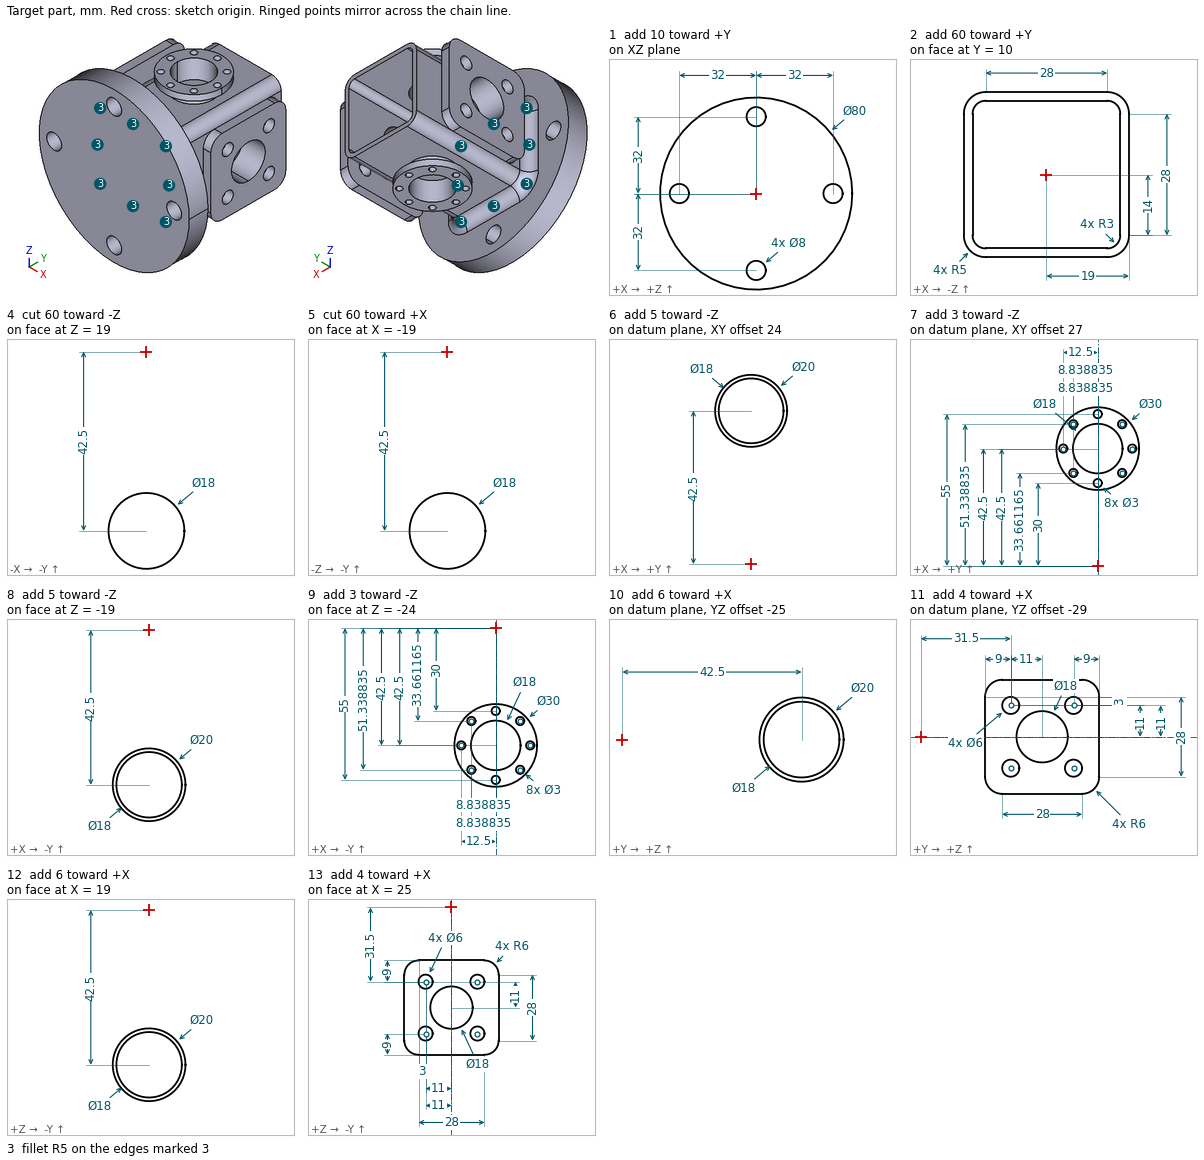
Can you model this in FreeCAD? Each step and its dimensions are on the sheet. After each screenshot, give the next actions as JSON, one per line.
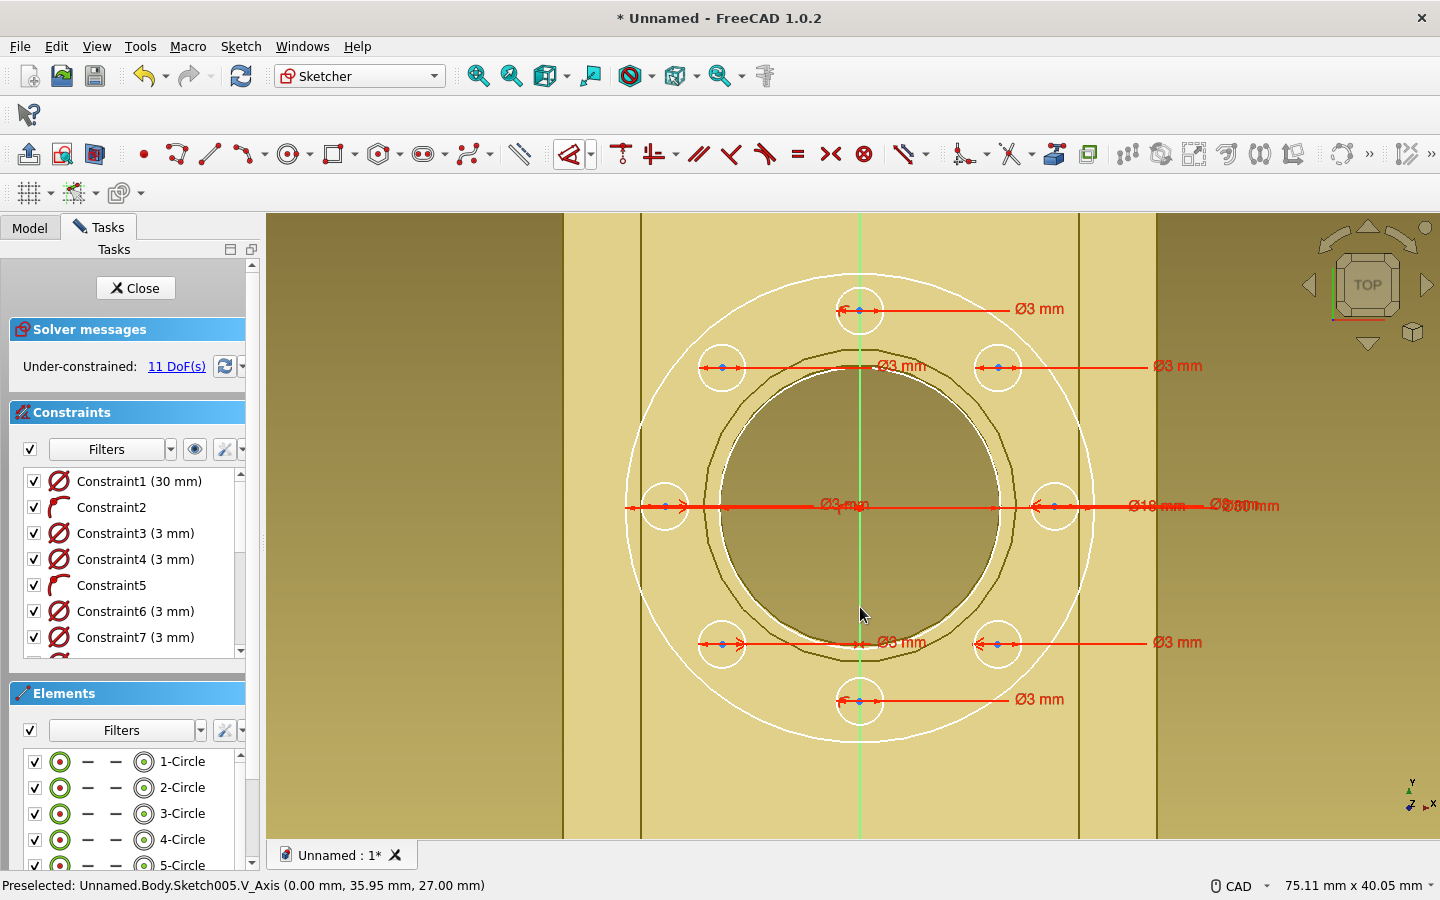
{"action": "left_click", "coordinate": [722, 368]}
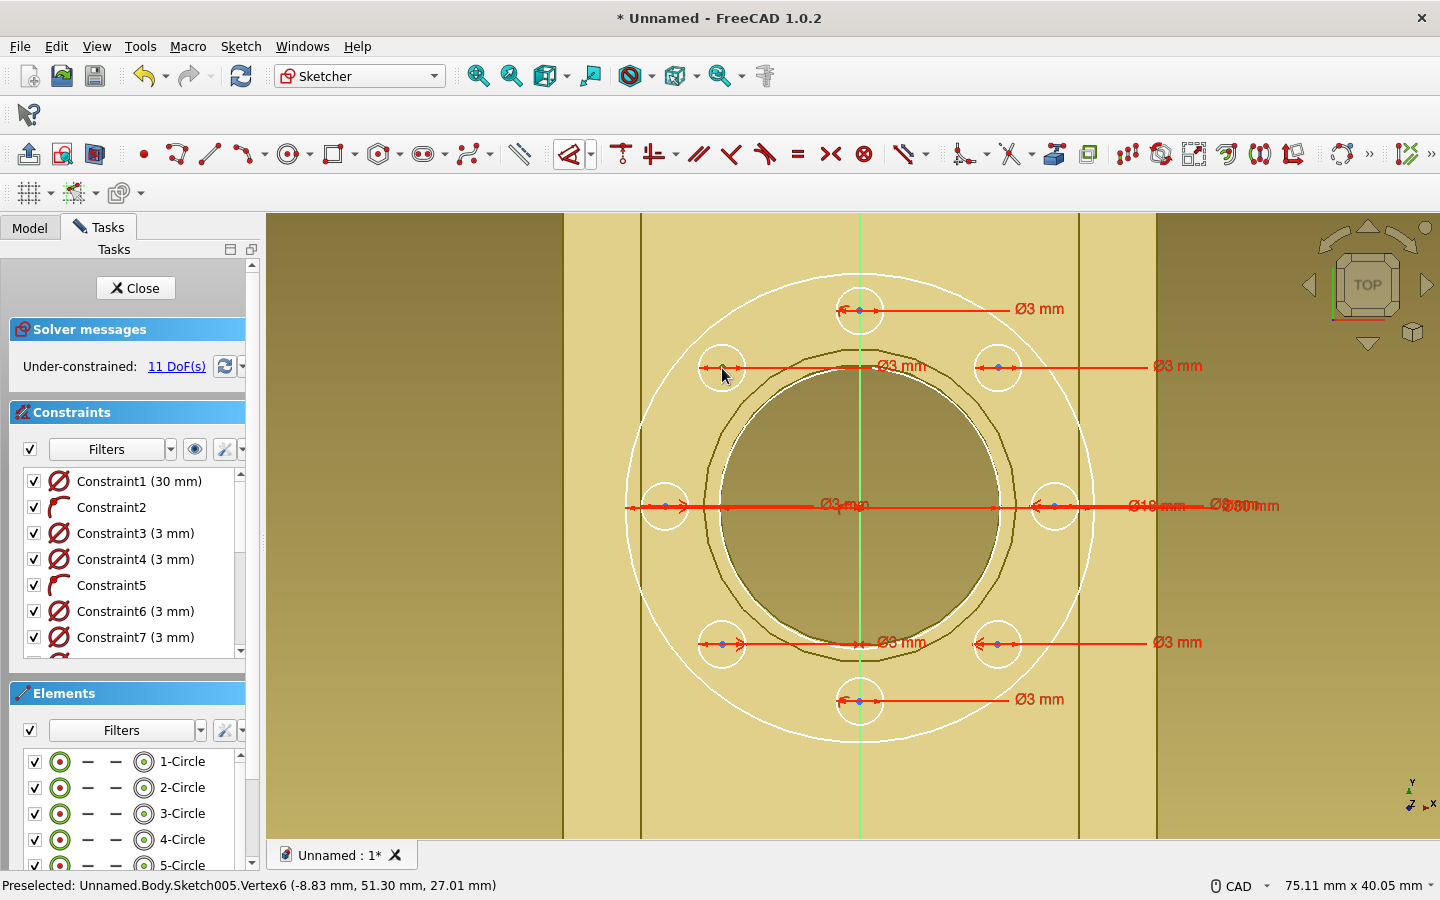
{"action": "left_click", "coordinate": [998, 368]}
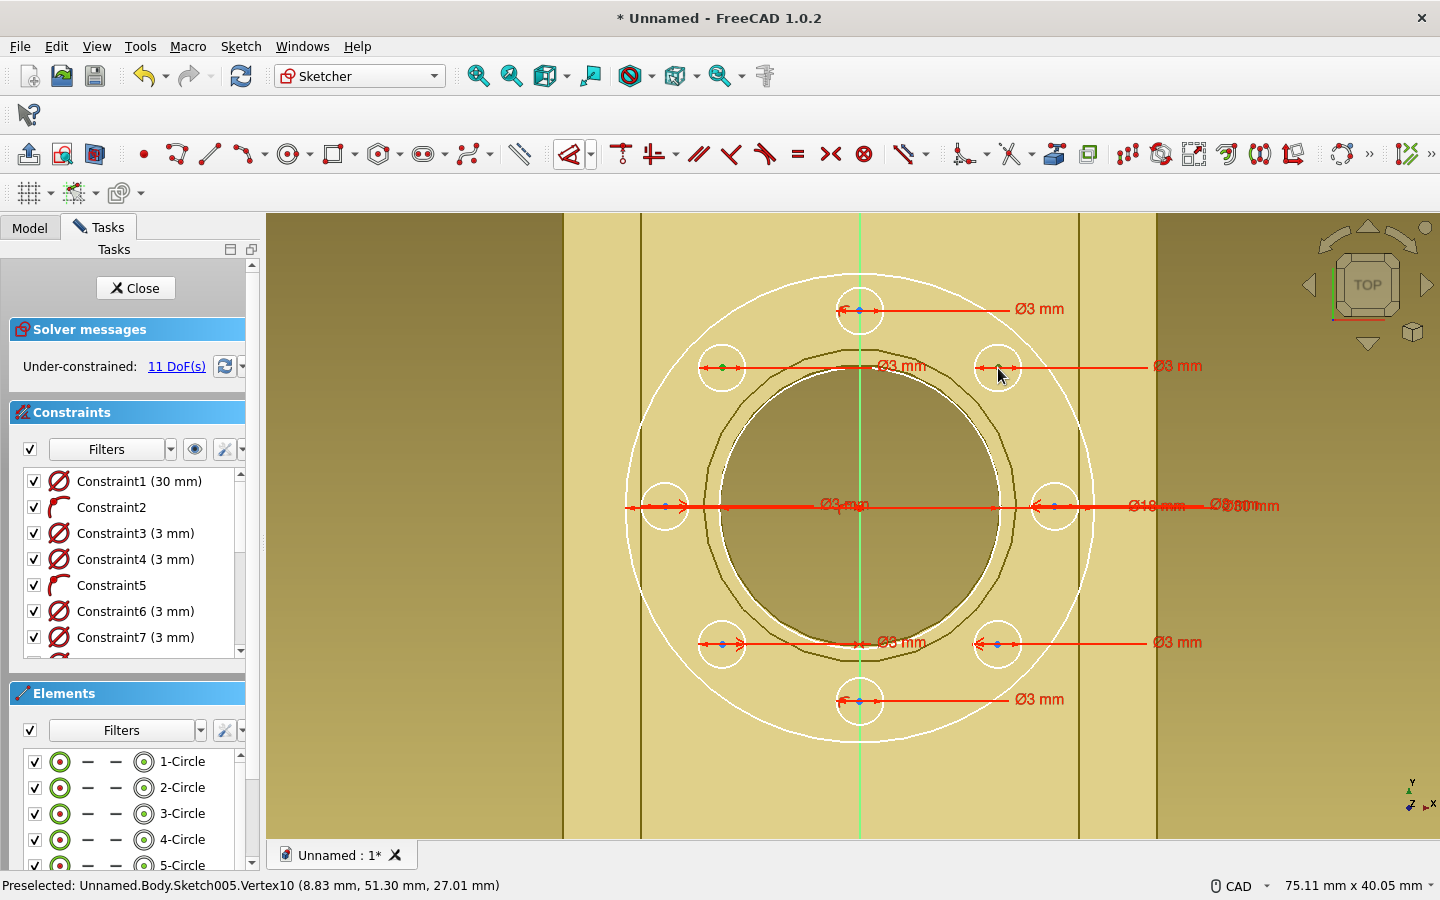
{"action": "left_click", "coordinate": [860, 607]}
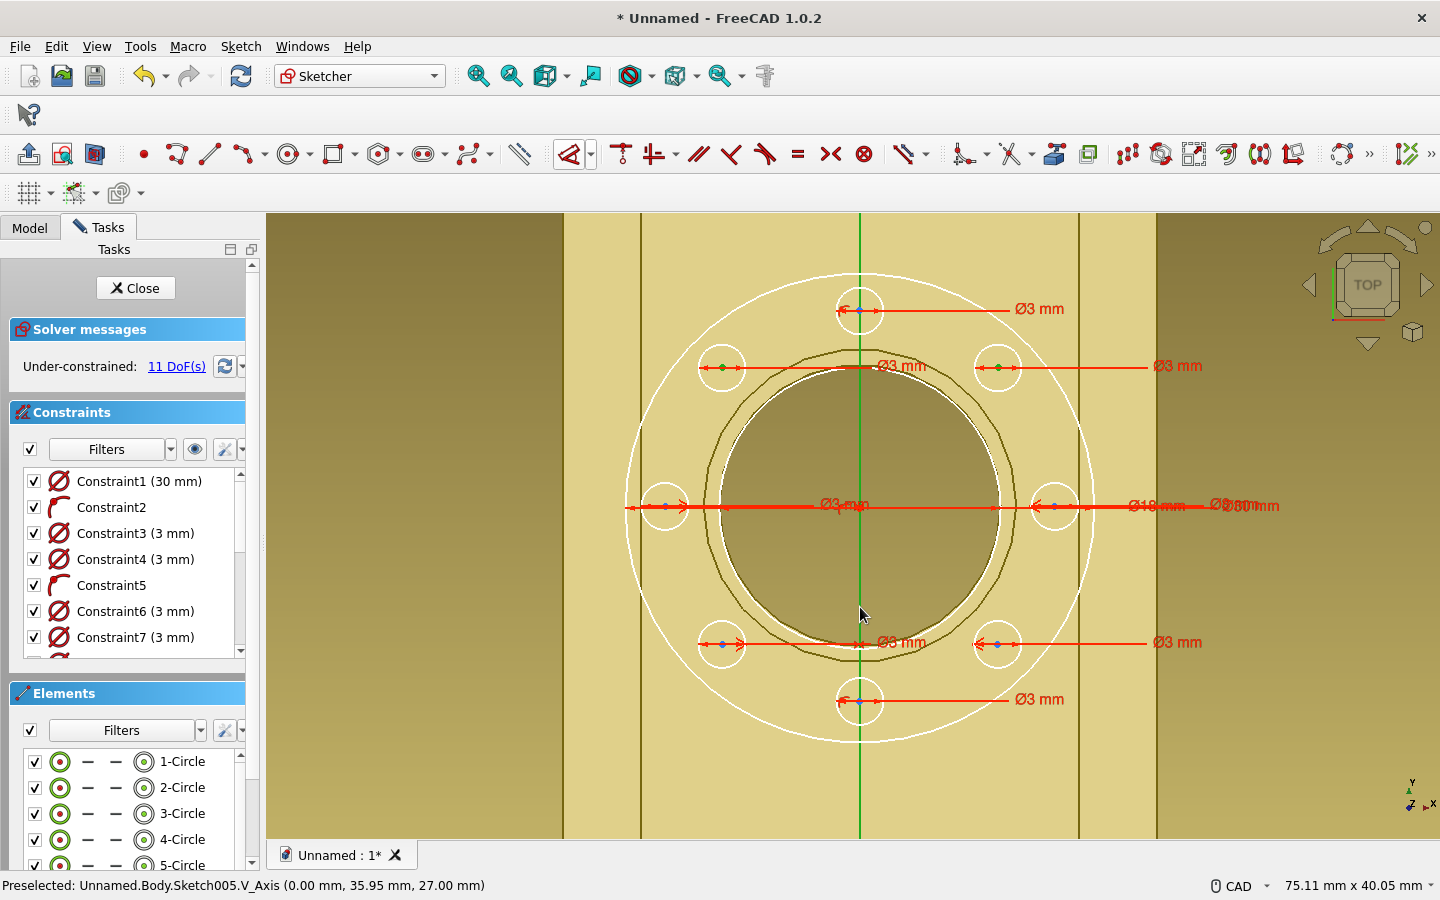
{"action": "left_click", "coordinate": [831, 154]}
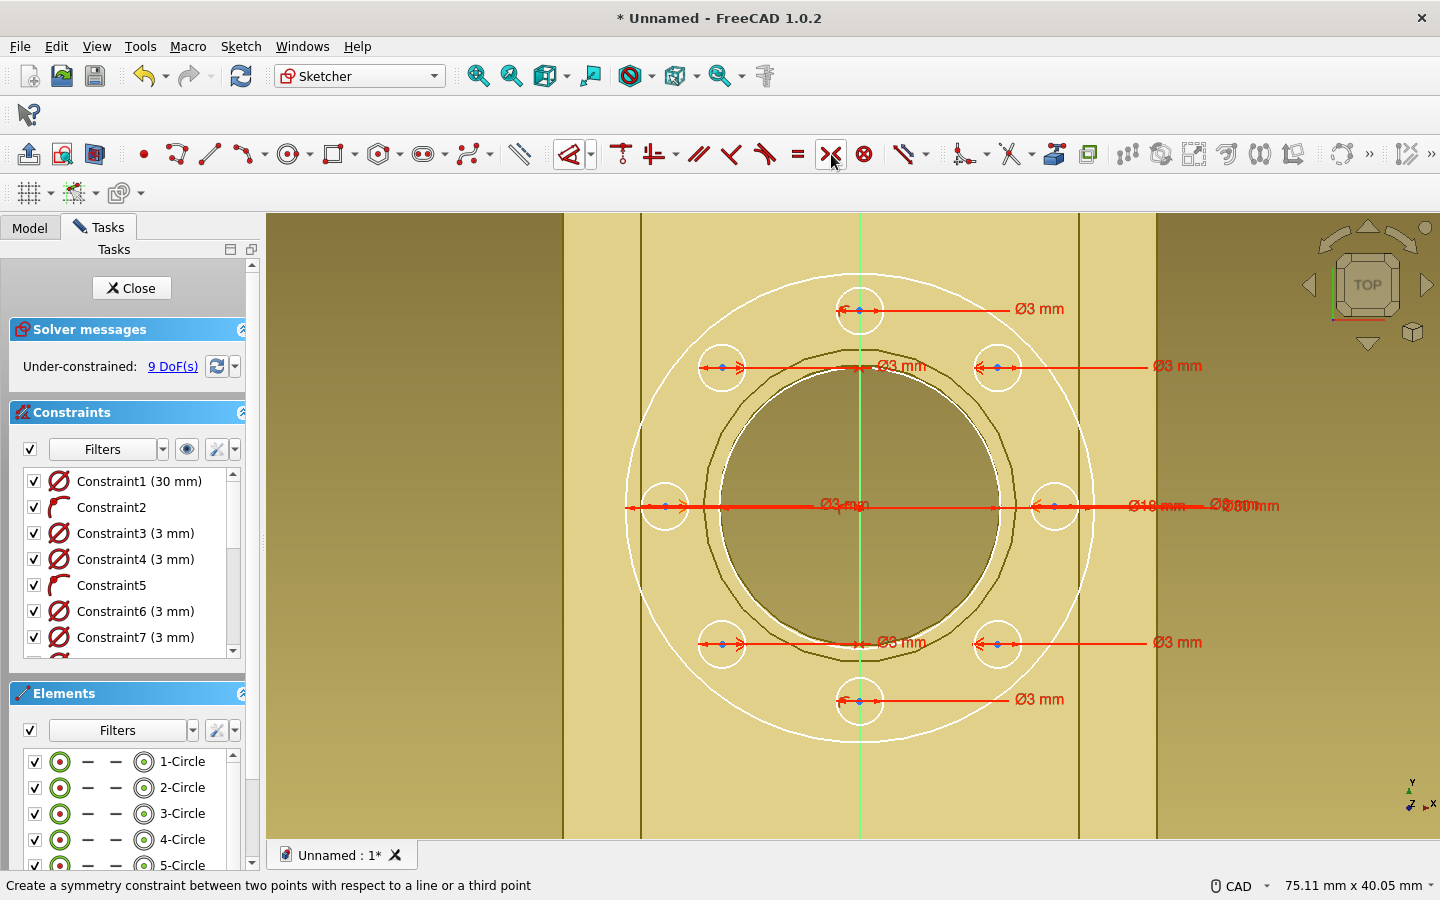
{"action": "left_click", "coordinate": [860, 701]}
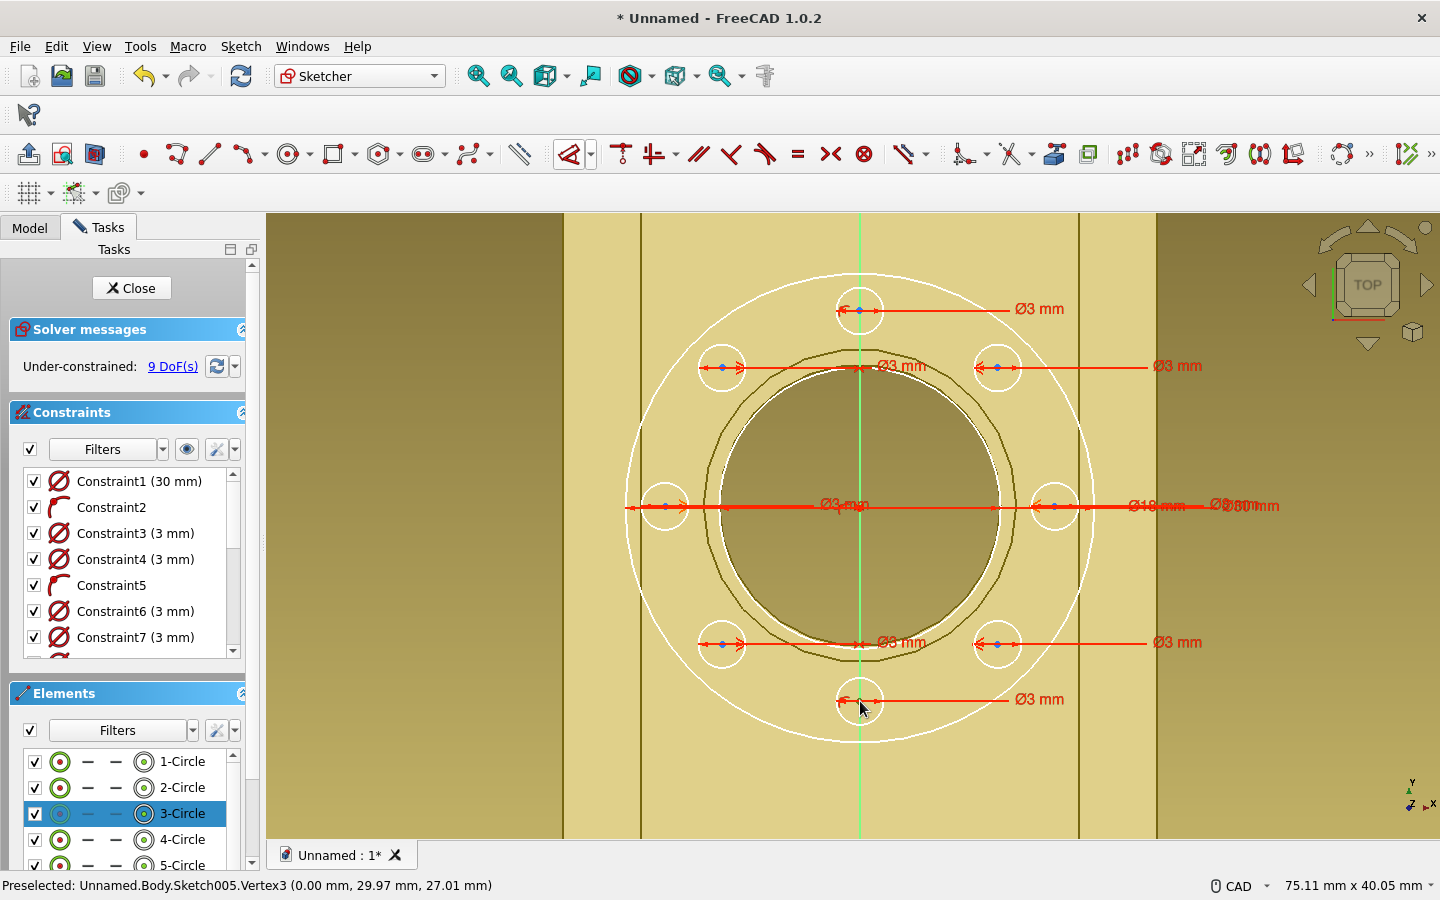
{"action": "key", "text": "i"}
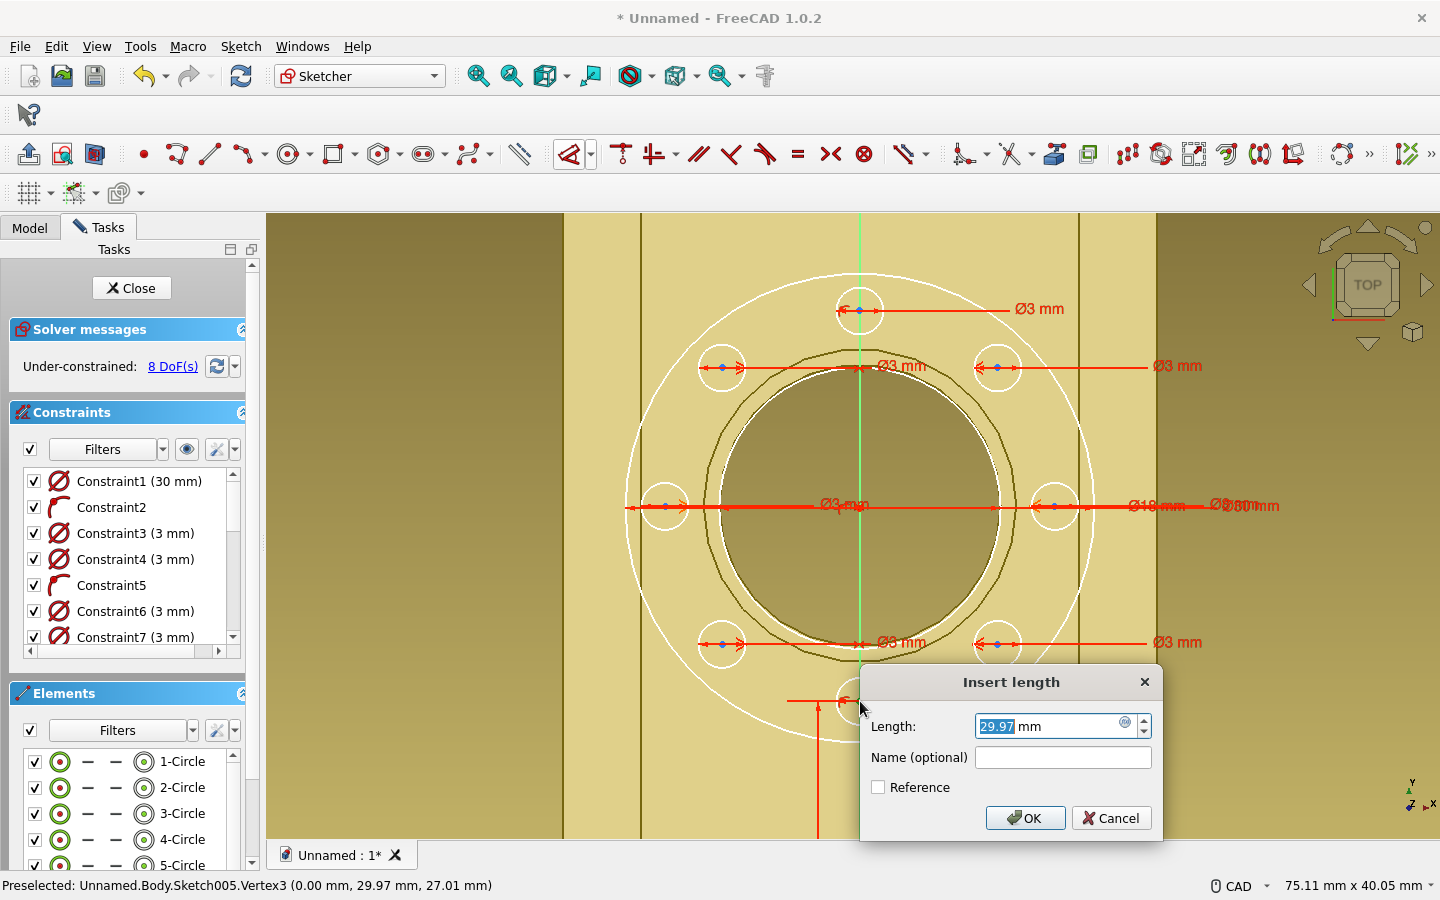
{"action": "type", "text": "30"}
{"action": "key", "text": "Return"}